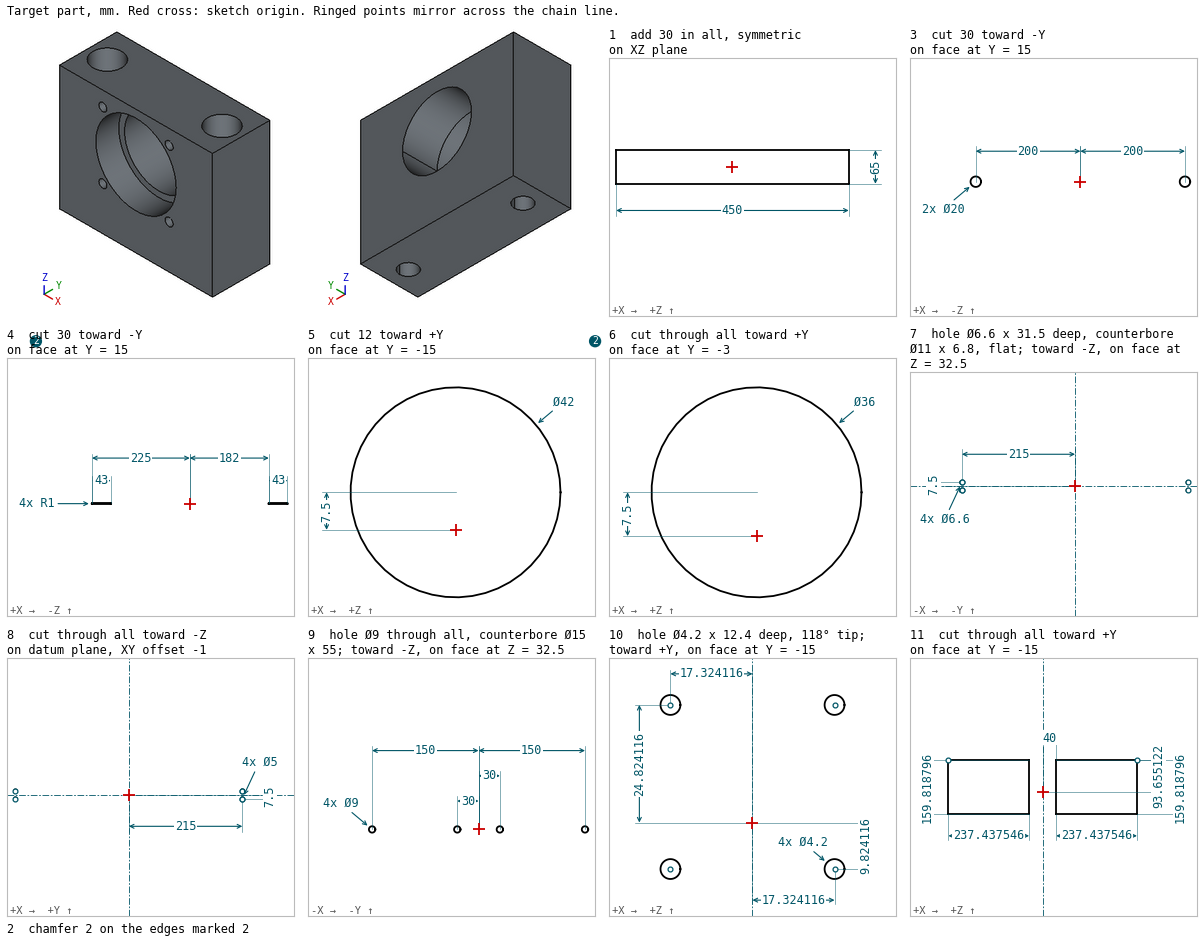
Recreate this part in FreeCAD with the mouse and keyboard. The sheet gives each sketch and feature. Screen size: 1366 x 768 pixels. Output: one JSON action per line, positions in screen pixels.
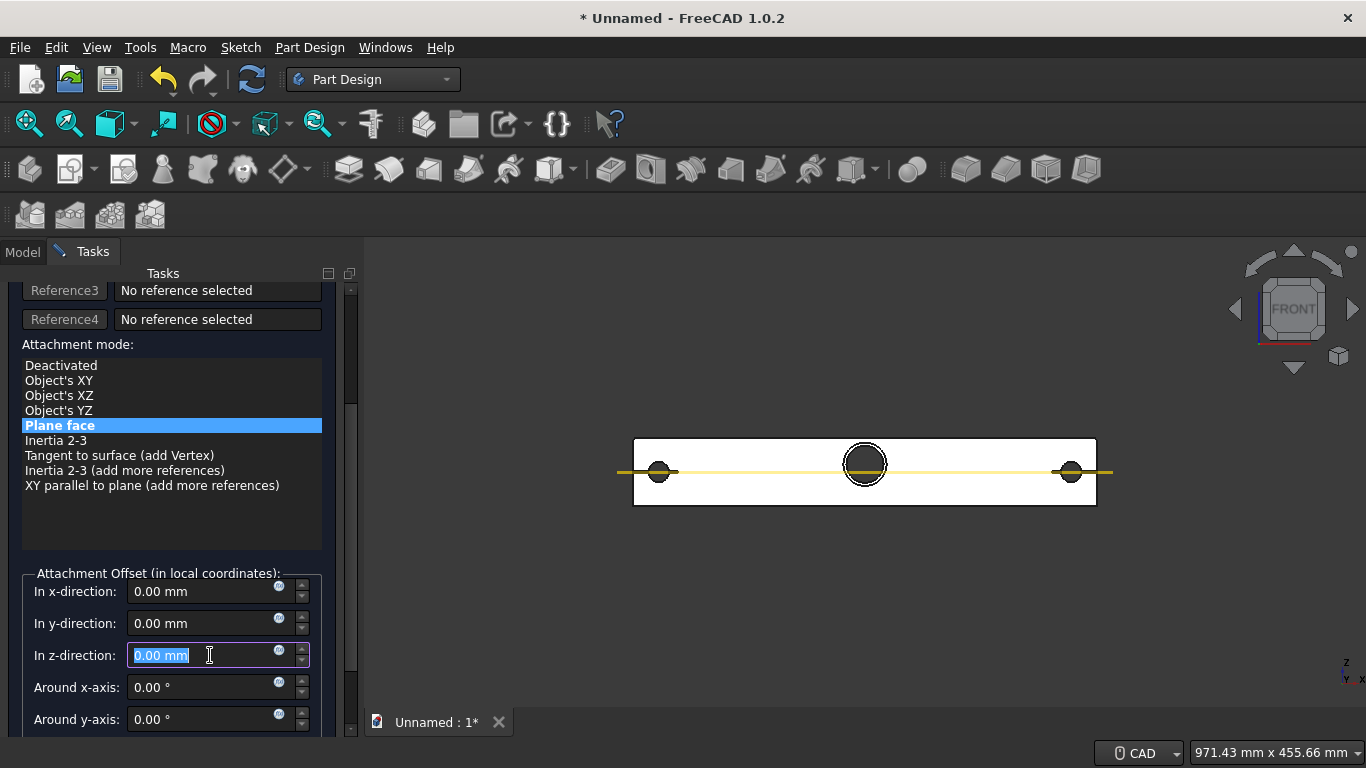
{"action": "type", "text": "-1"}
{"action": "key", "text": "Tab"}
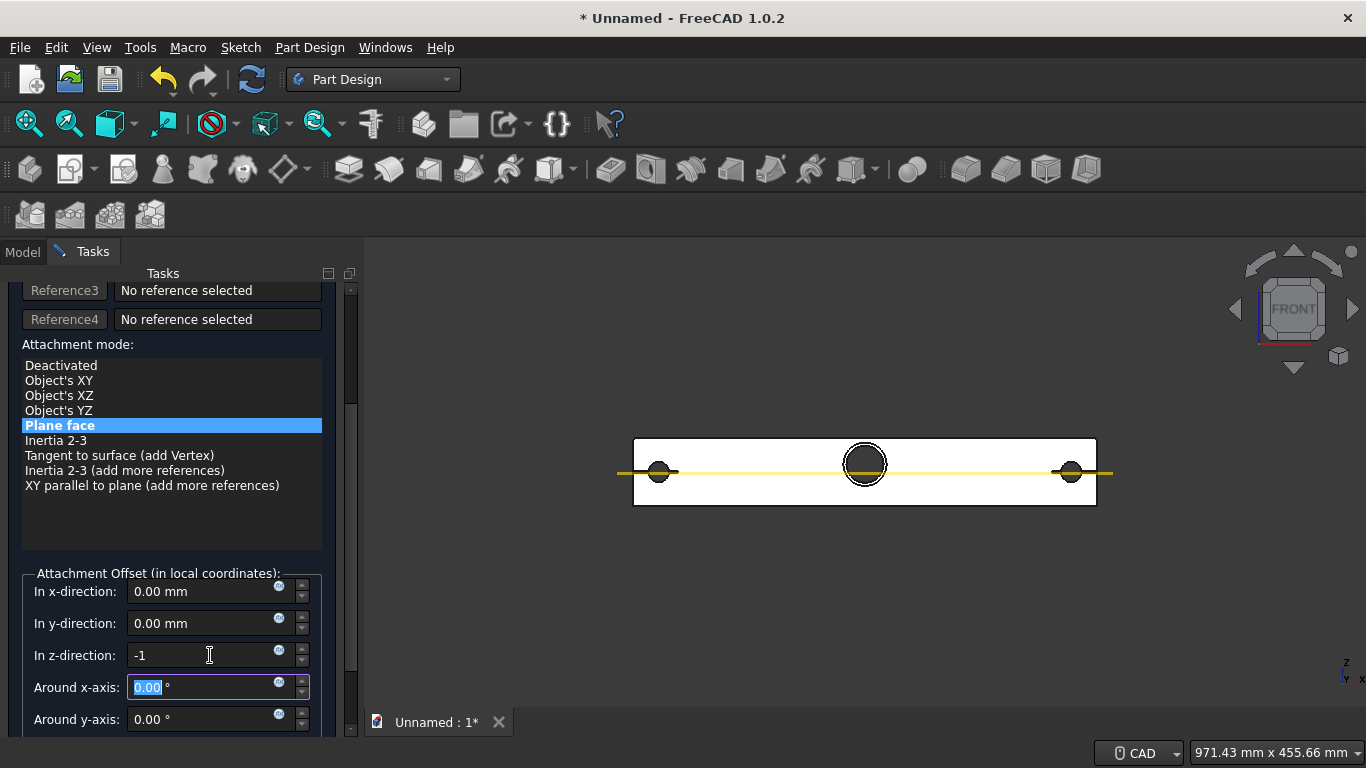
{"action": "scroll", "coordinate": [351, 510], "scroll_direction": "up", "scroll_amount": 4}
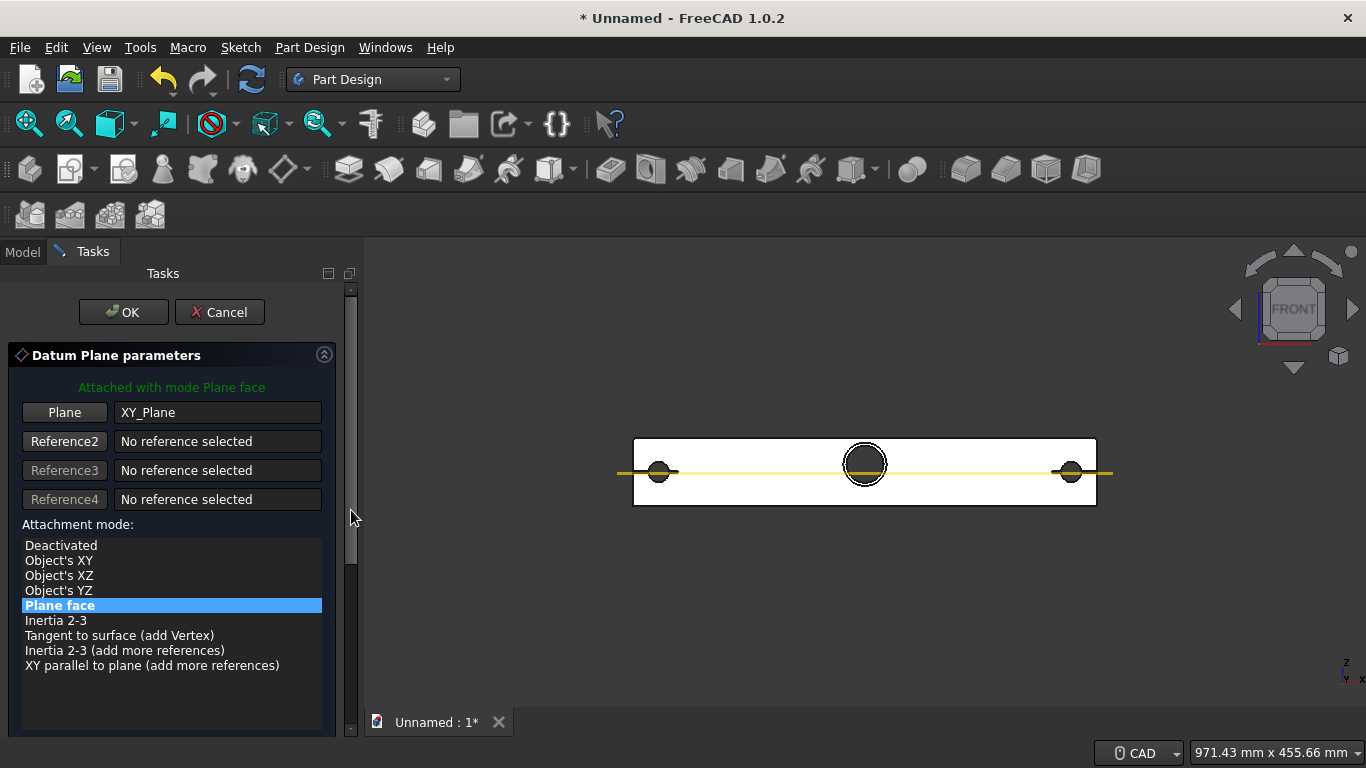
{"action": "left_click", "coordinate": [124, 312]}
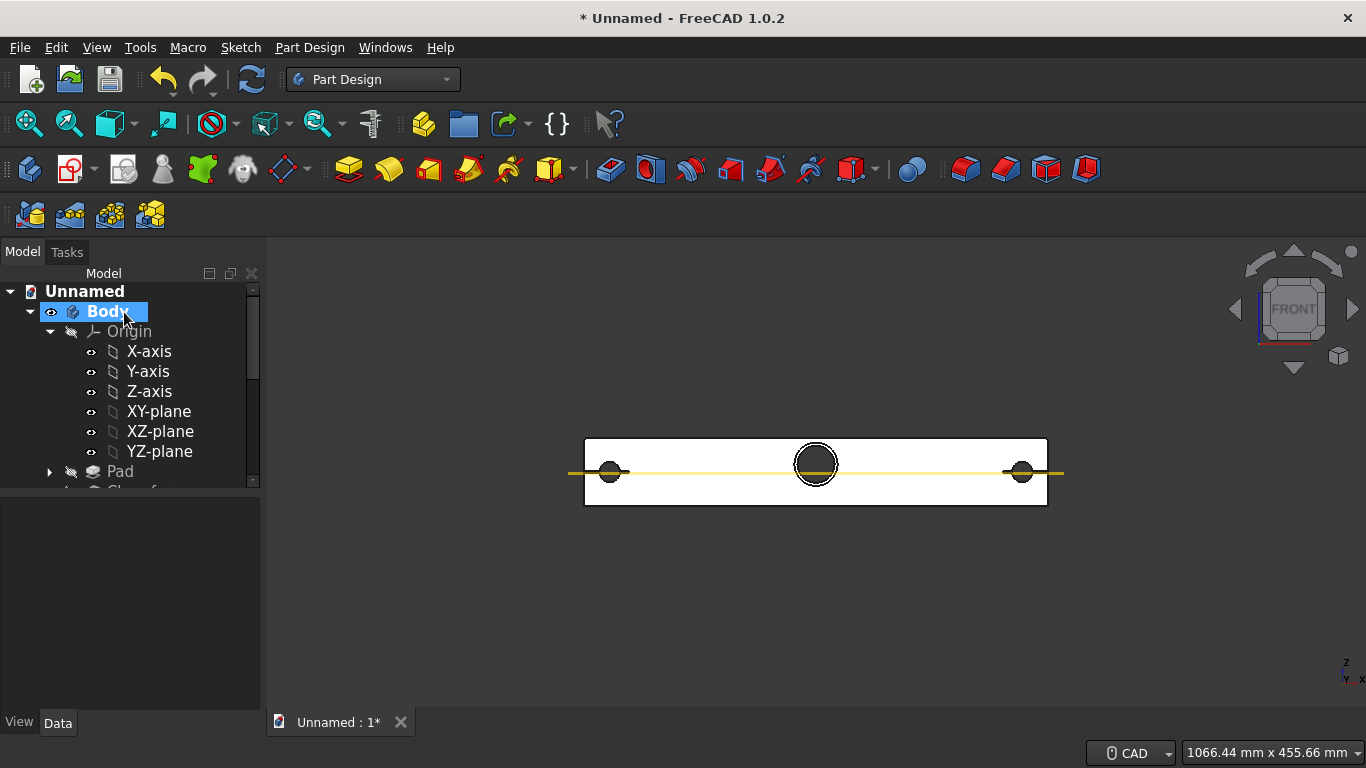
{"action": "scroll", "coordinate": [100, 387], "scroll_direction": "down", "scroll_amount": 3}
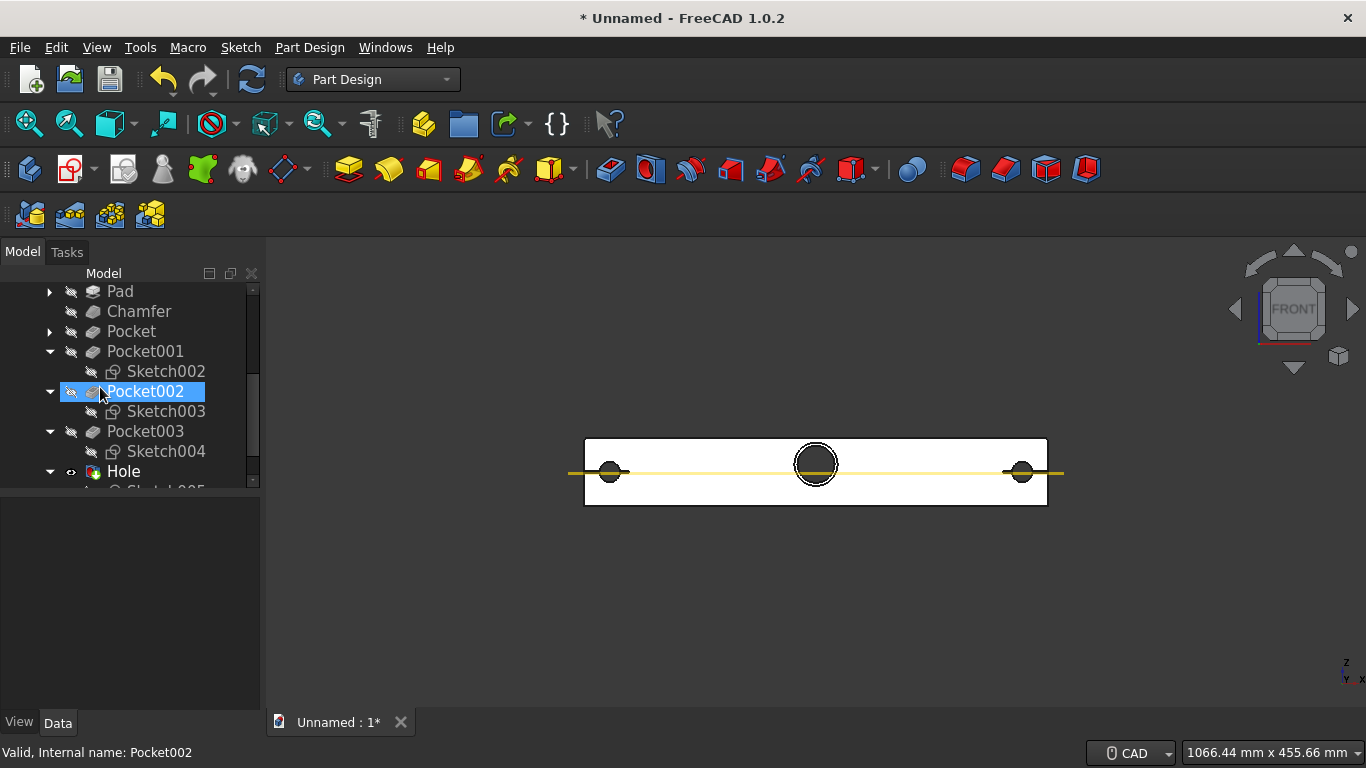
{"action": "scroll", "coordinate": [140, 387], "scroll_direction": "up", "scroll_amount": 15}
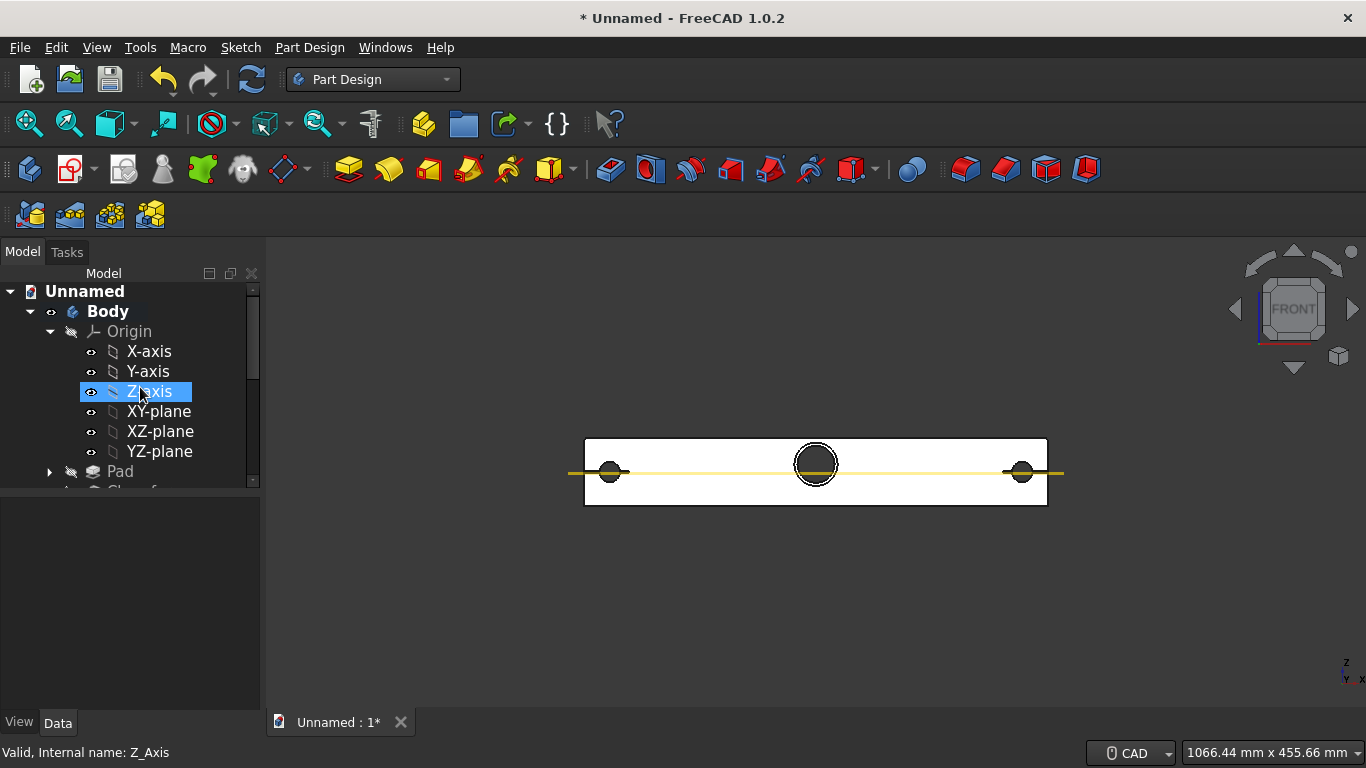
{"action": "scroll", "coordinate": [100, 387], "scroll_direction": "down", "scroll_amount": 6}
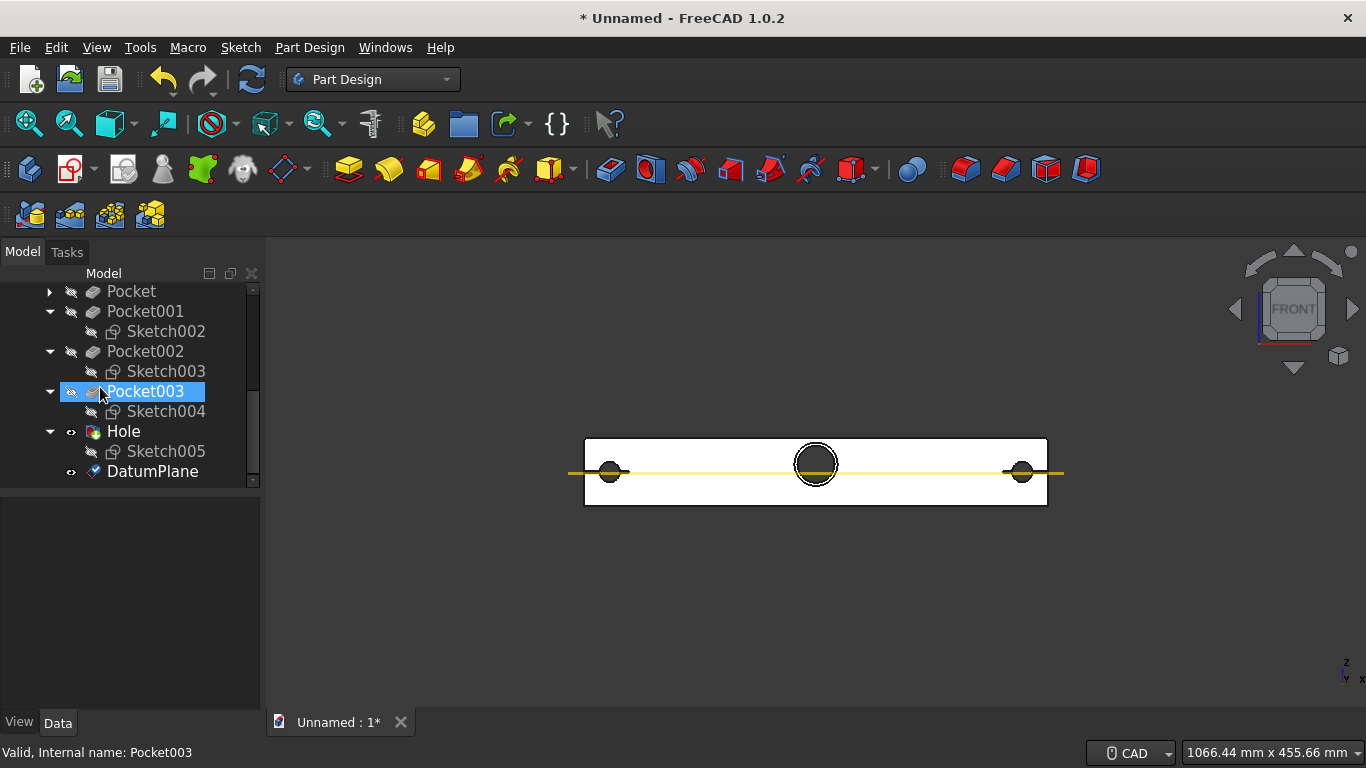
{"action": "left_click", "coordinate": [116, 472]}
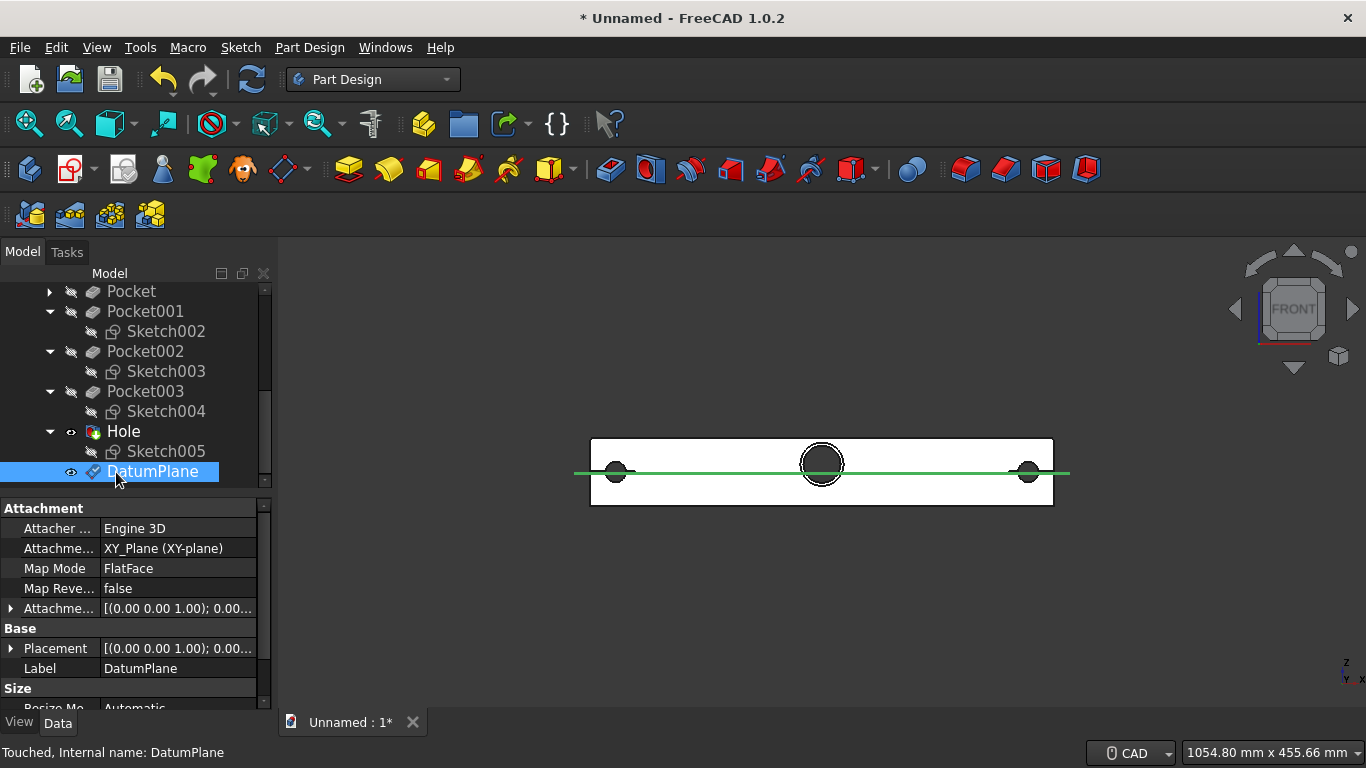
{"action": "left_click", "coordinate": [70, 170]}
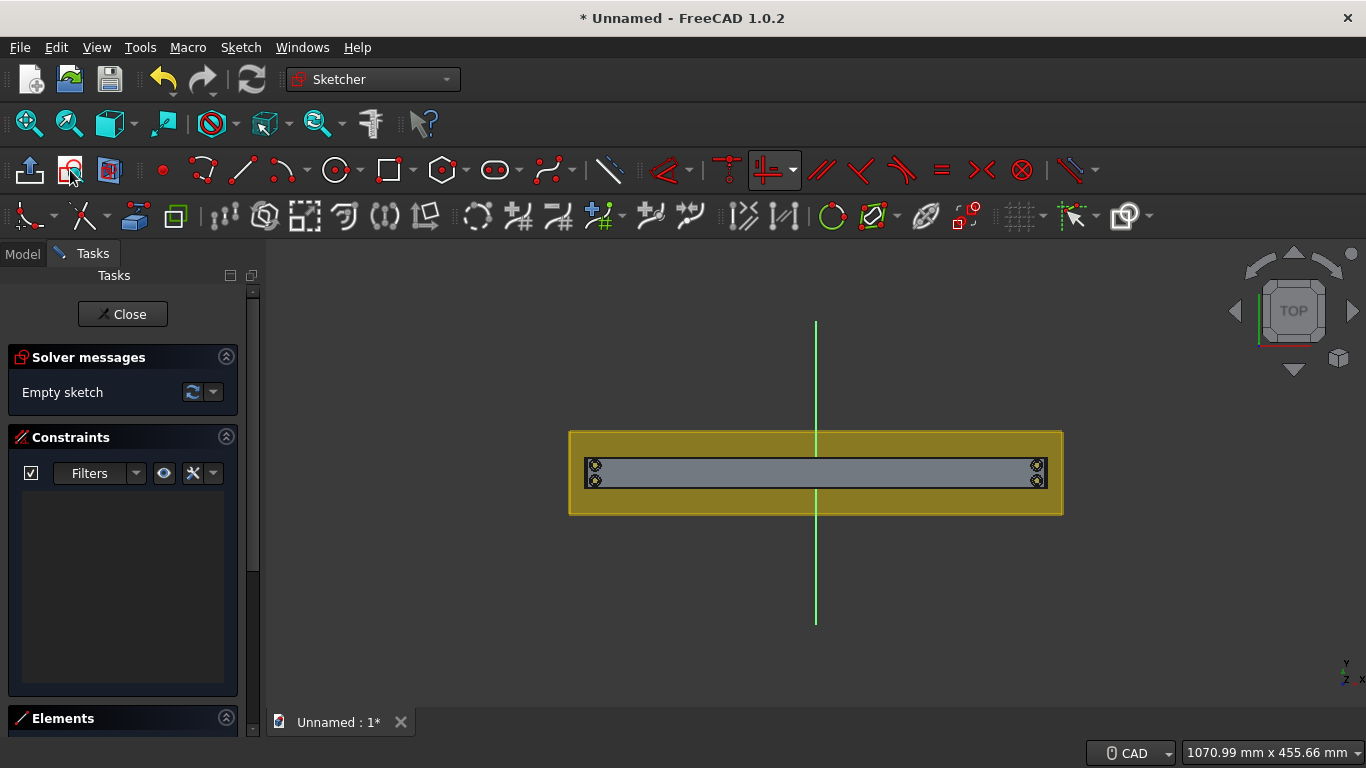
{"action": "key", "text": "q s"}